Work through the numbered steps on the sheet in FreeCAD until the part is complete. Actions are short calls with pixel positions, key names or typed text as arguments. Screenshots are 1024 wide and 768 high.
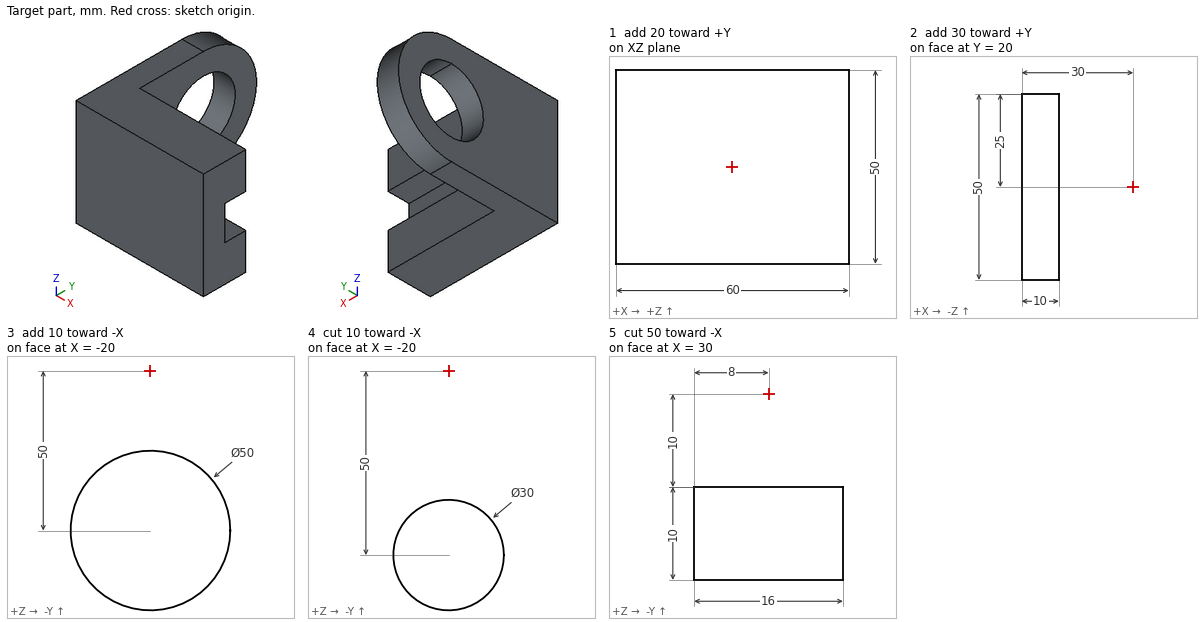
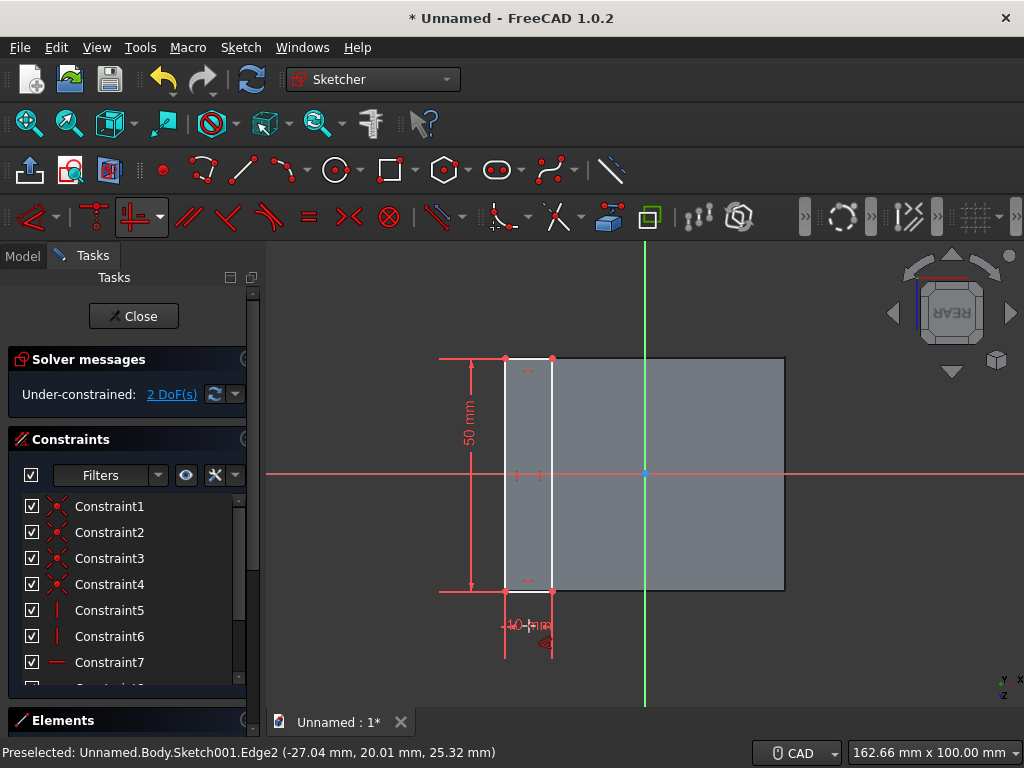
click(505, 359)
click(575, 325)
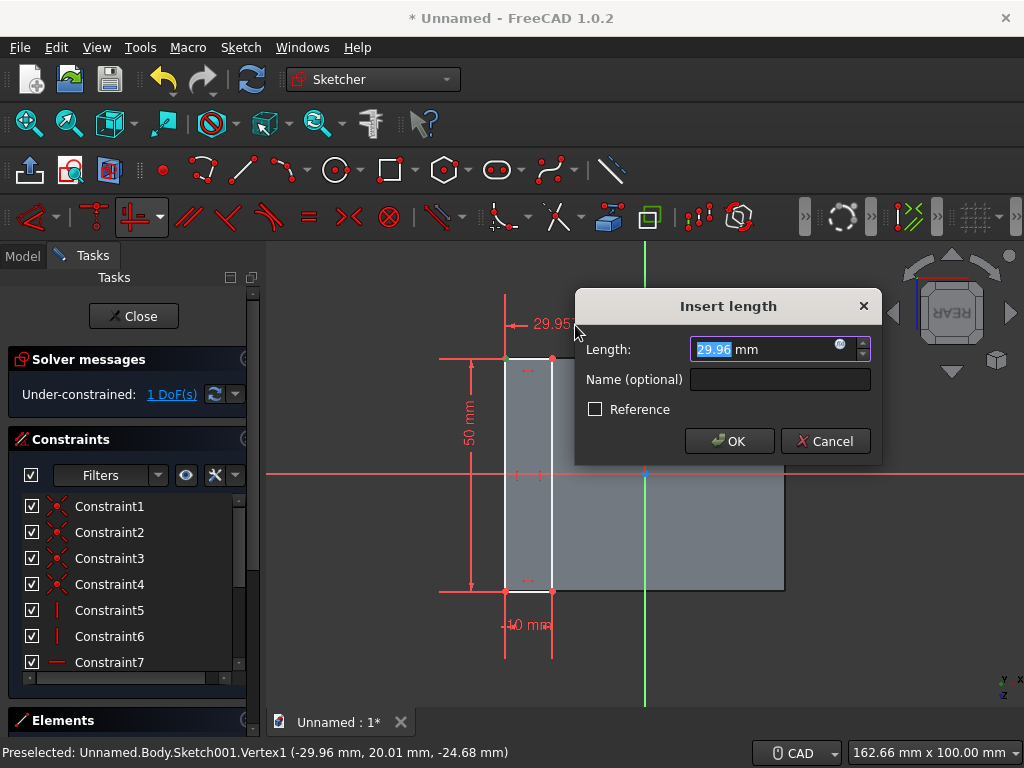
text(30)
key(Return)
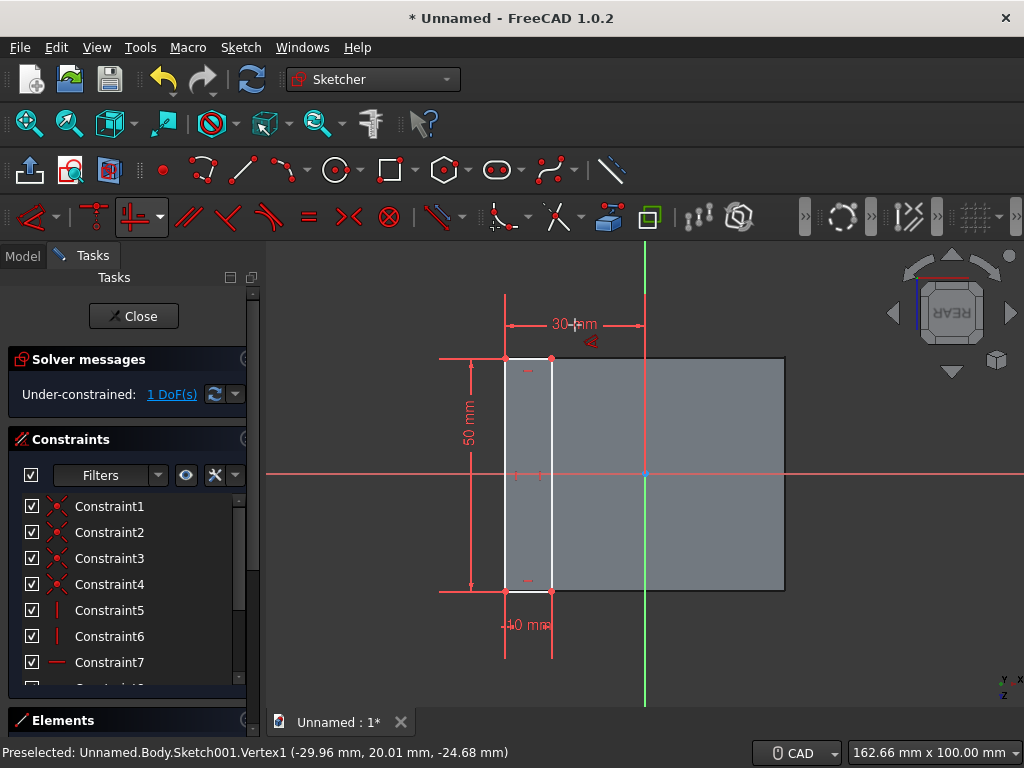
click(505, 359)
click(679, 417)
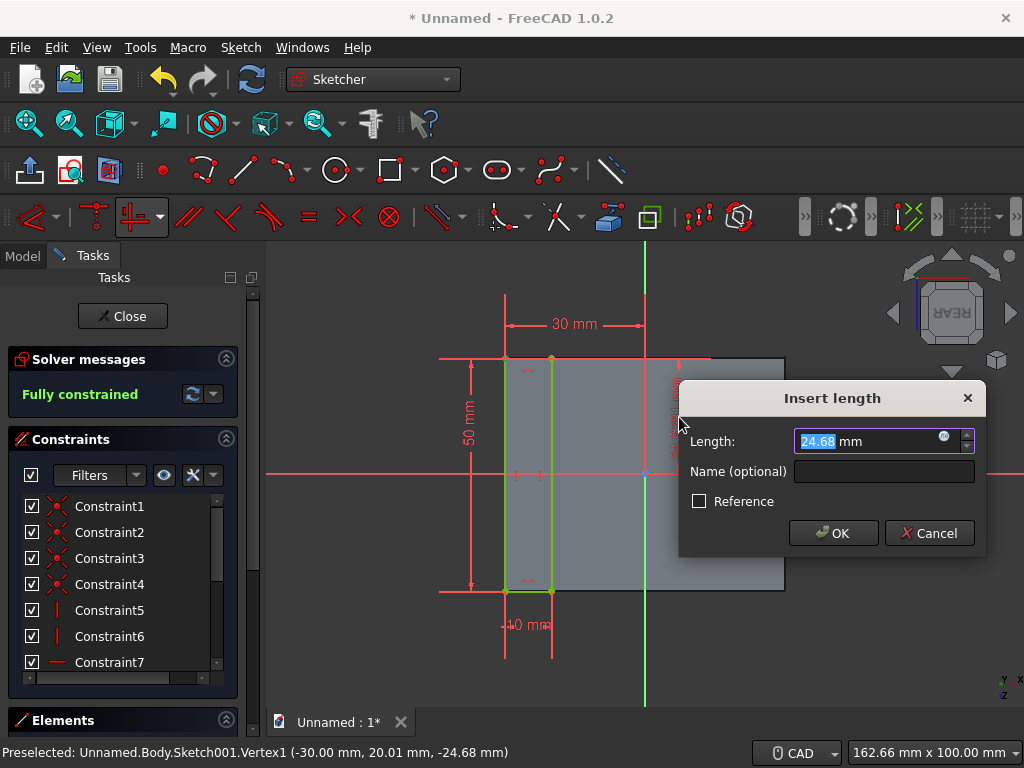
text(25)
key(Return)
key(Escape)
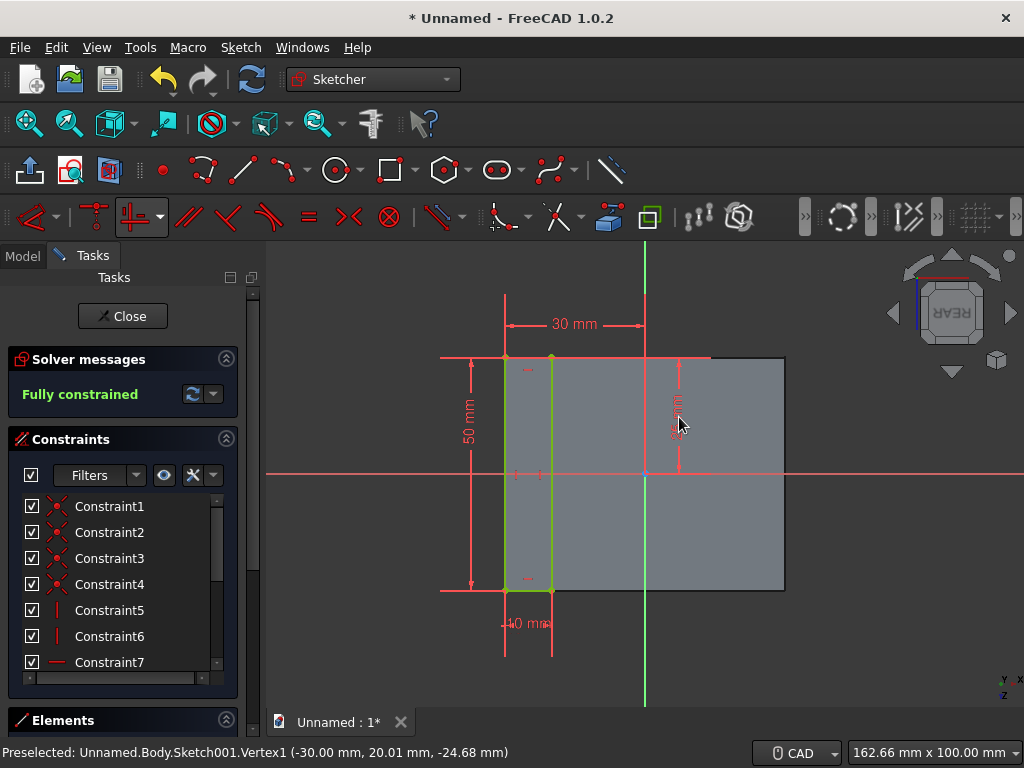
click(123, 316)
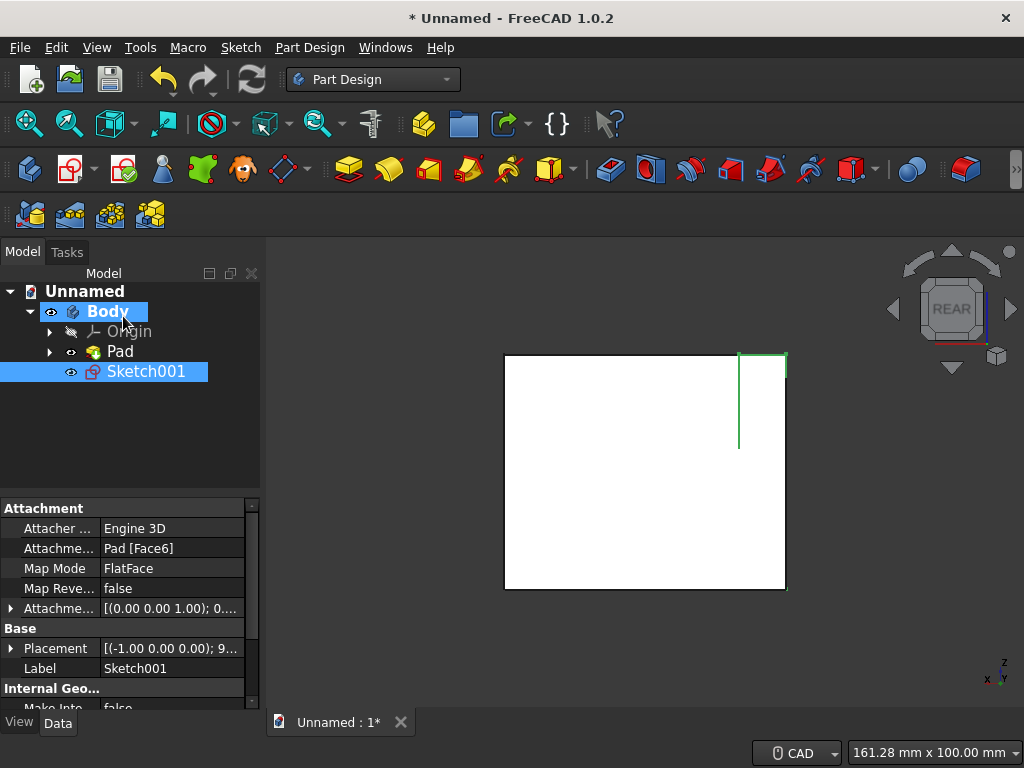
click(350, 170)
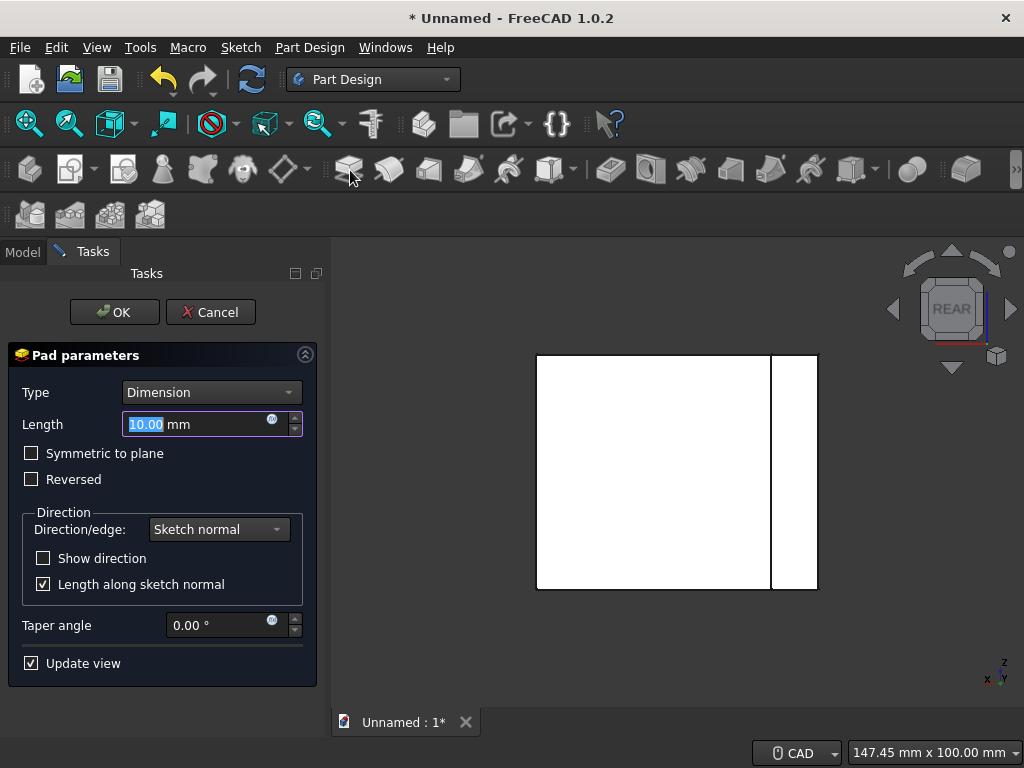
text(30)
key(Tab)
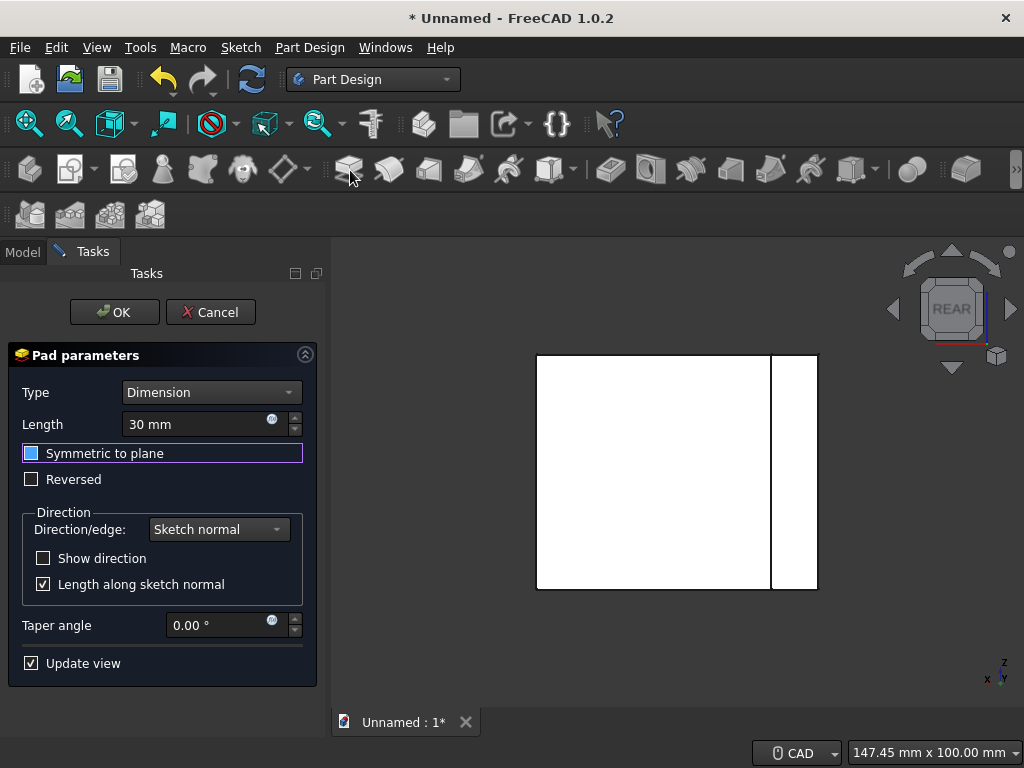
click(115, 312)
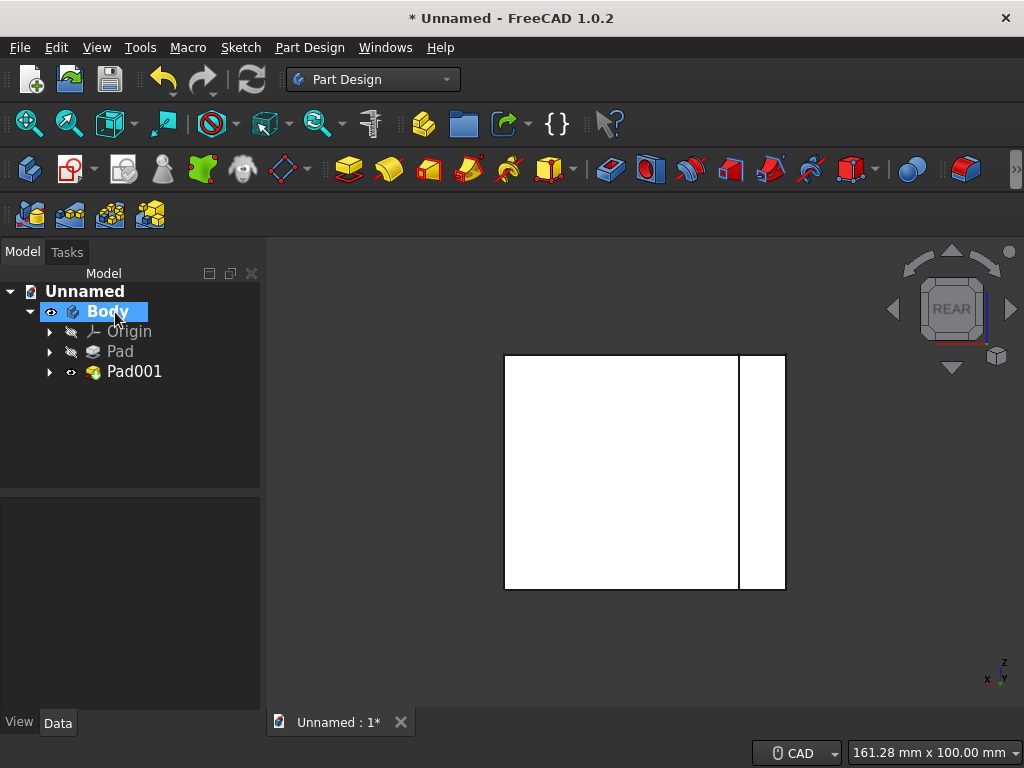
key(0)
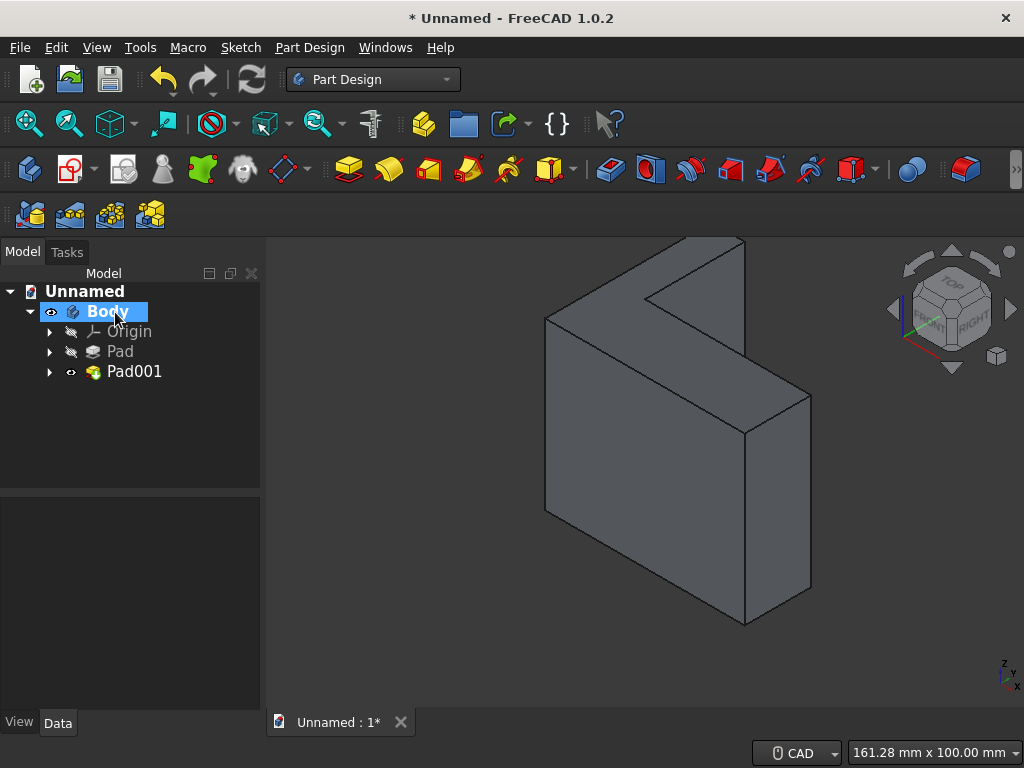
click(30, 124)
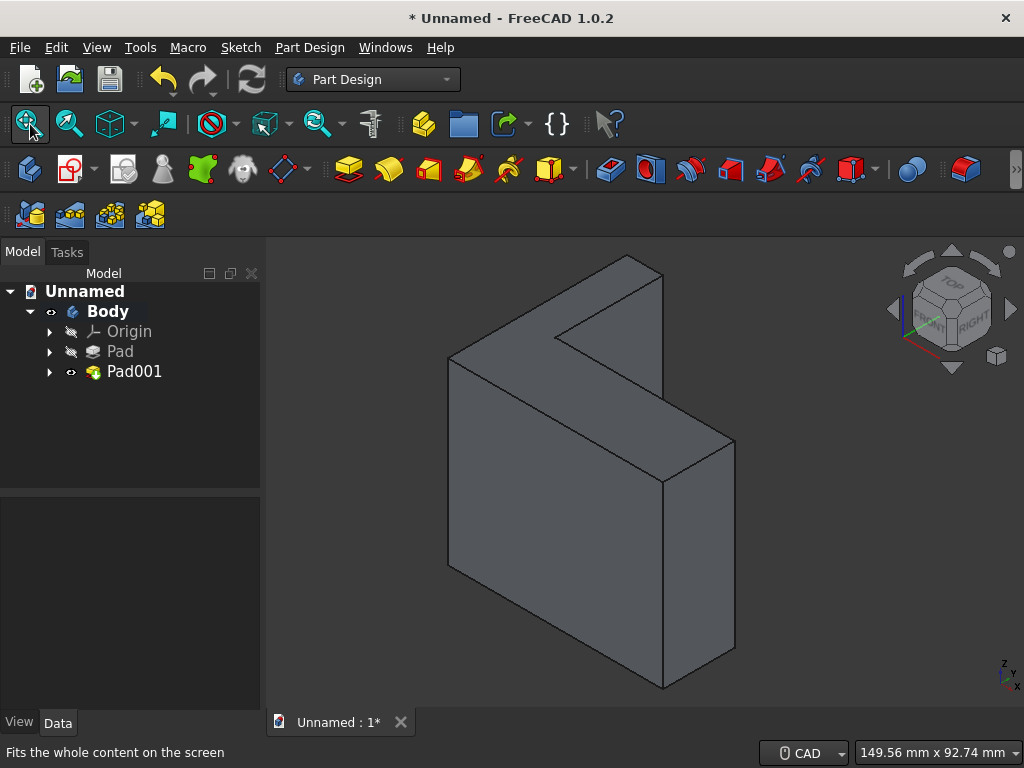
key(3)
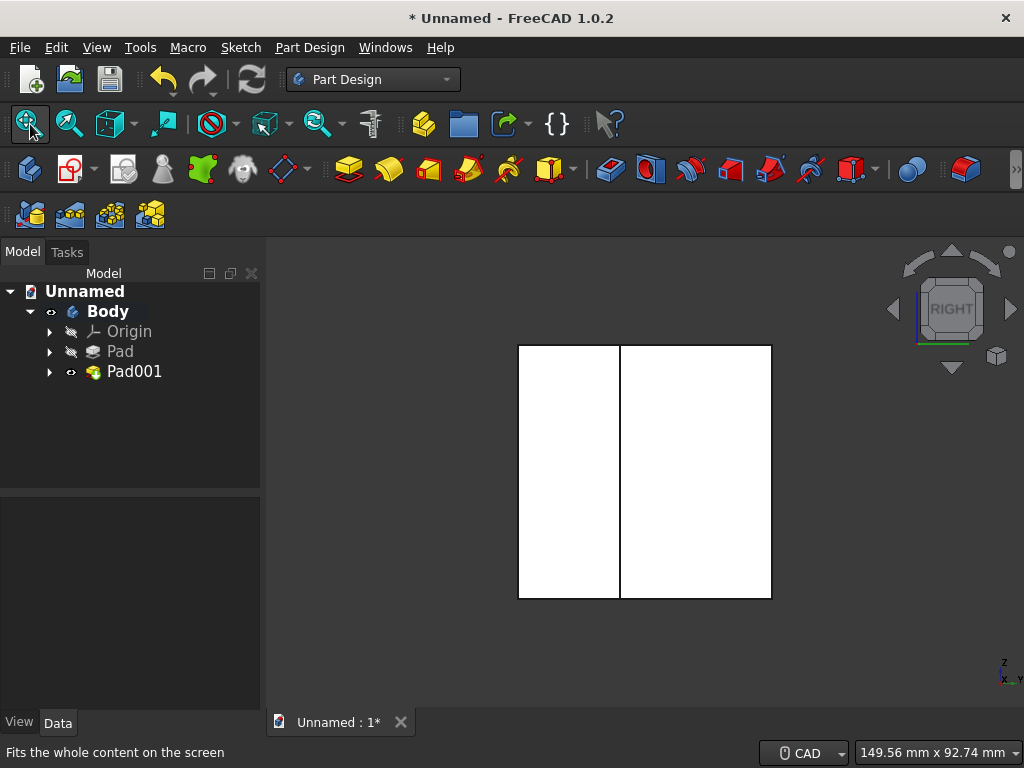
click(696, 435)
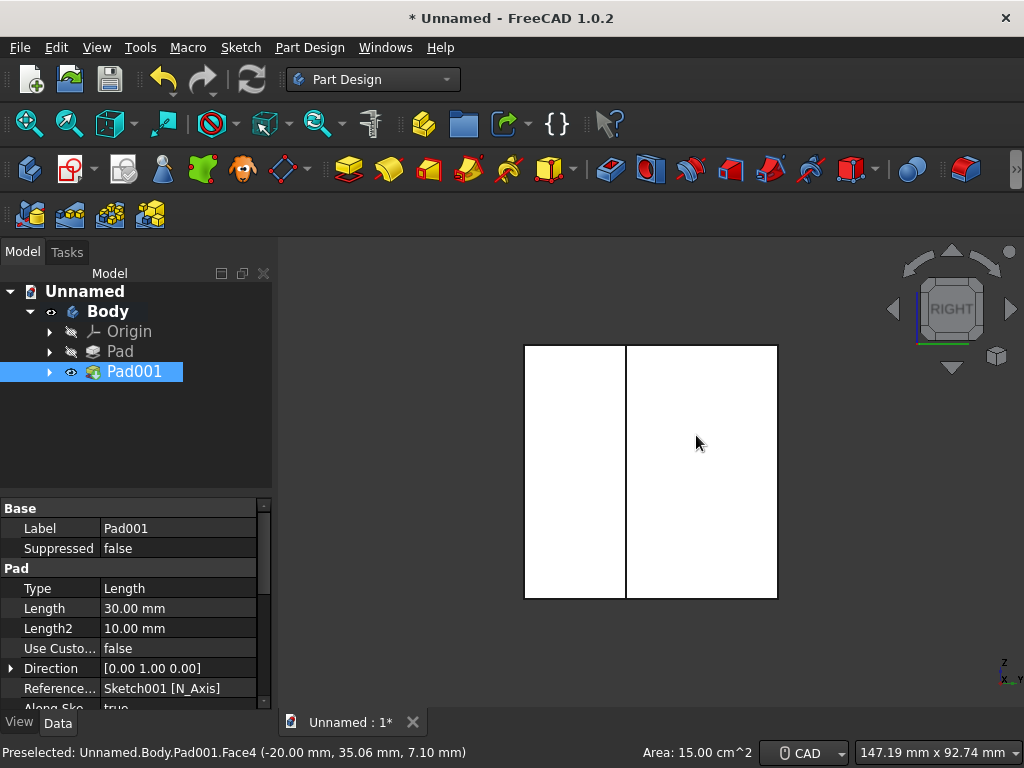
click(70, 170)